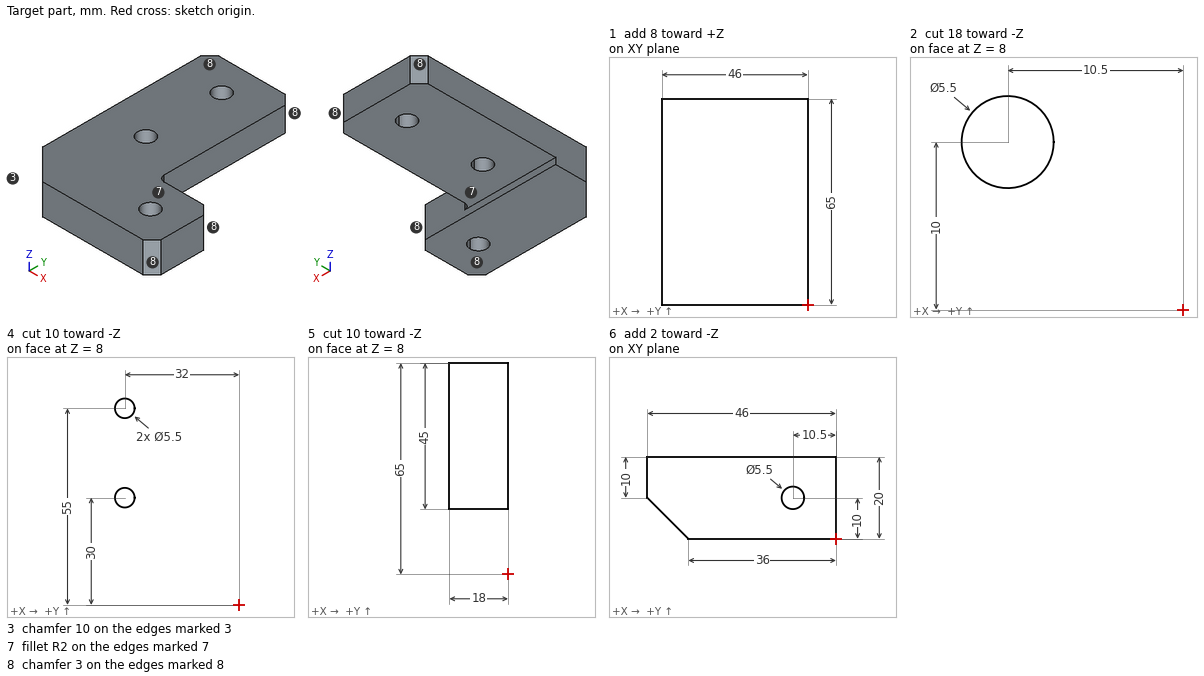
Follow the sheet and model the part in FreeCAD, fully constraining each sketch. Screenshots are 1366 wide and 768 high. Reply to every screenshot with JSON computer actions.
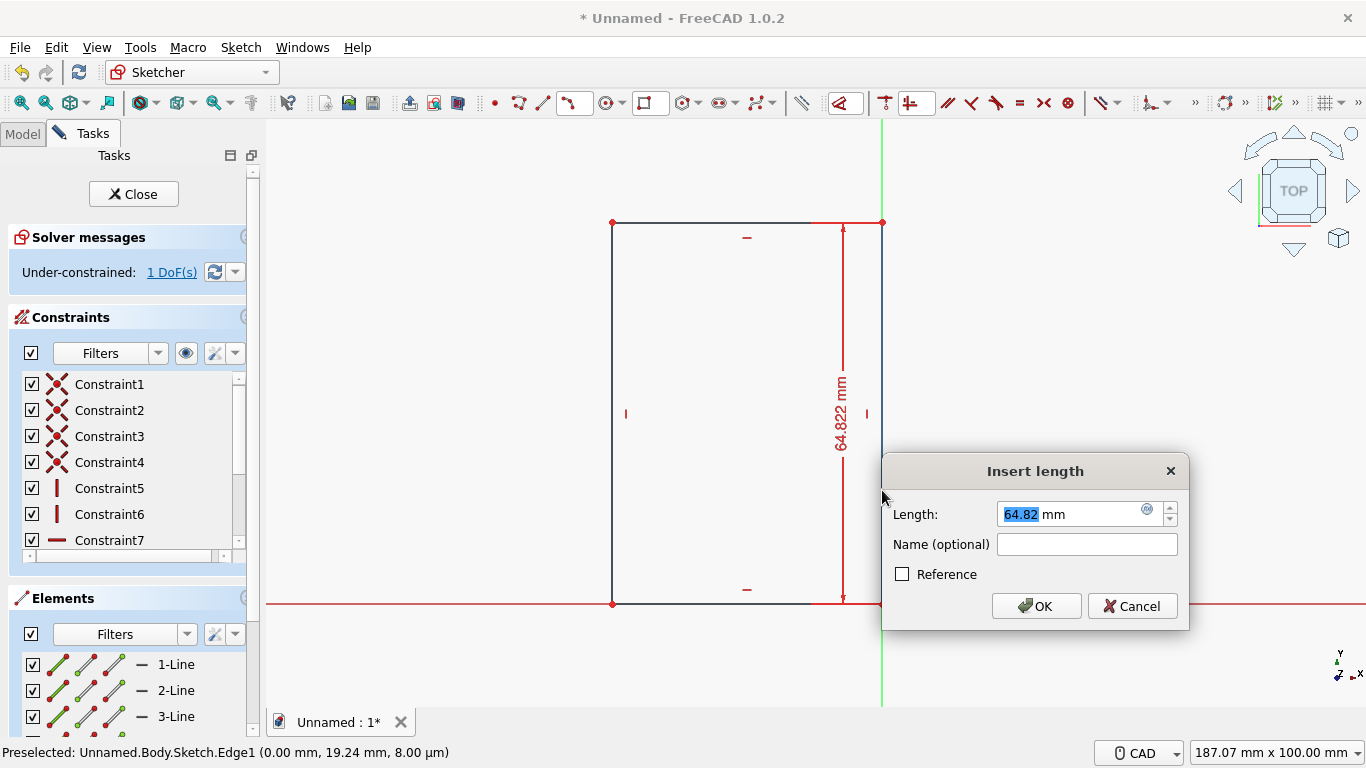
{"action": "type", "text": "65"}
{"action": "key", "text": "Return"}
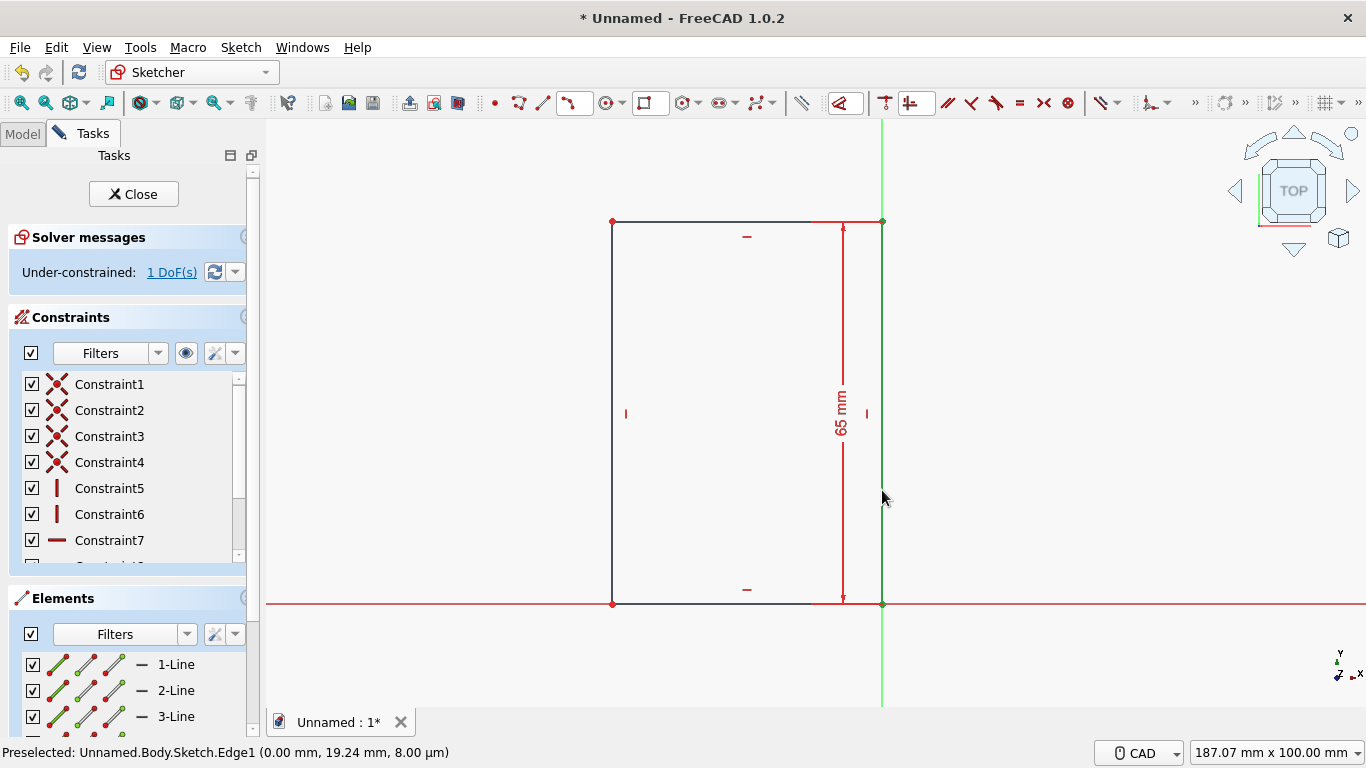
{"action": "left_click", "coordinate": [801, 222]}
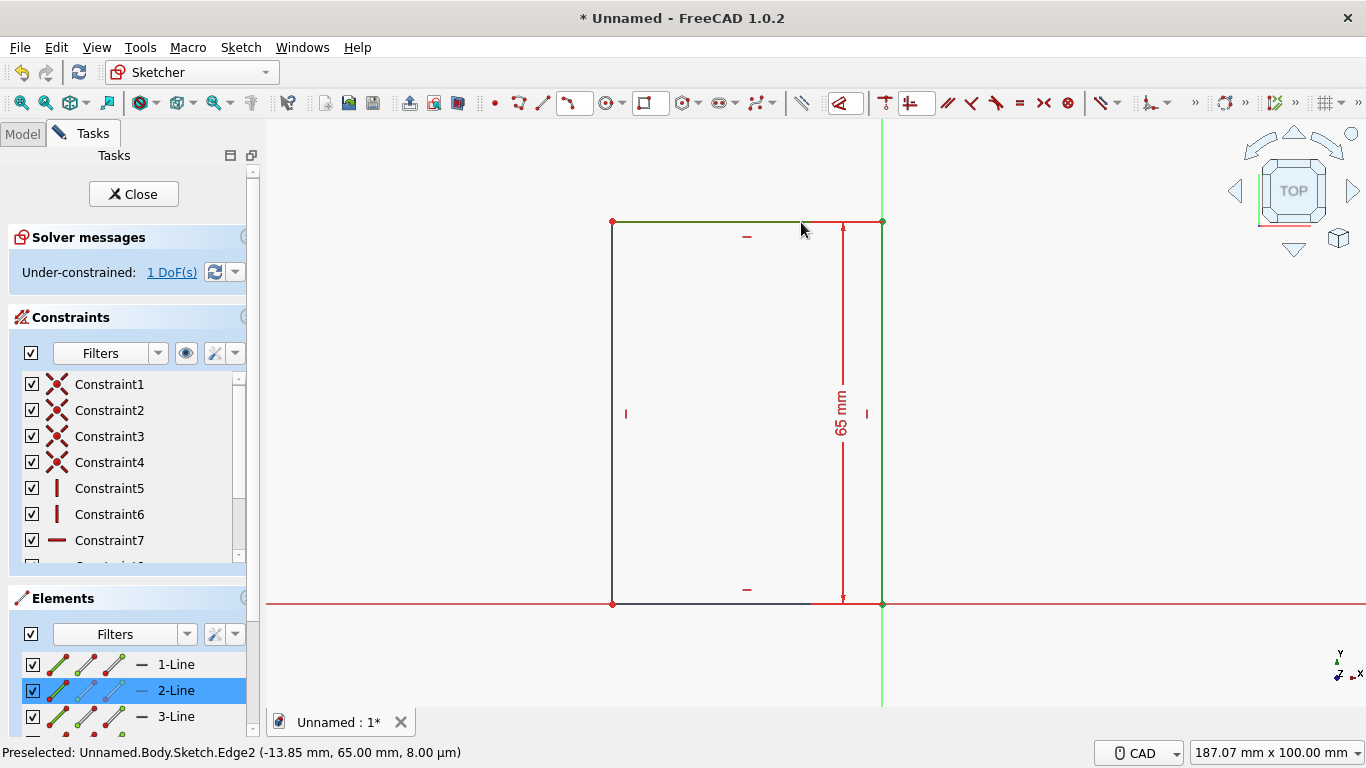
{"action": "key", "text": "l"}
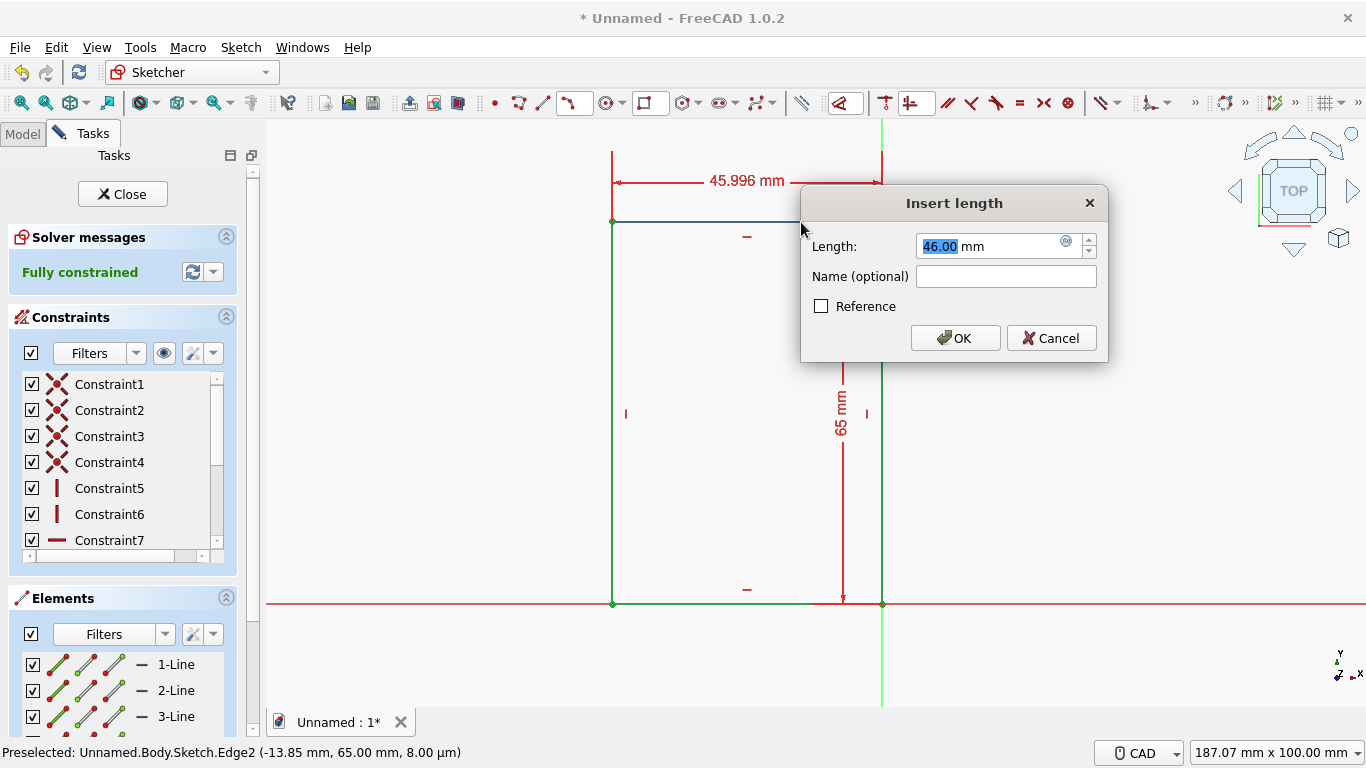
{"action": "type", "text": "46"}
{"action": "key", "text": "Return"}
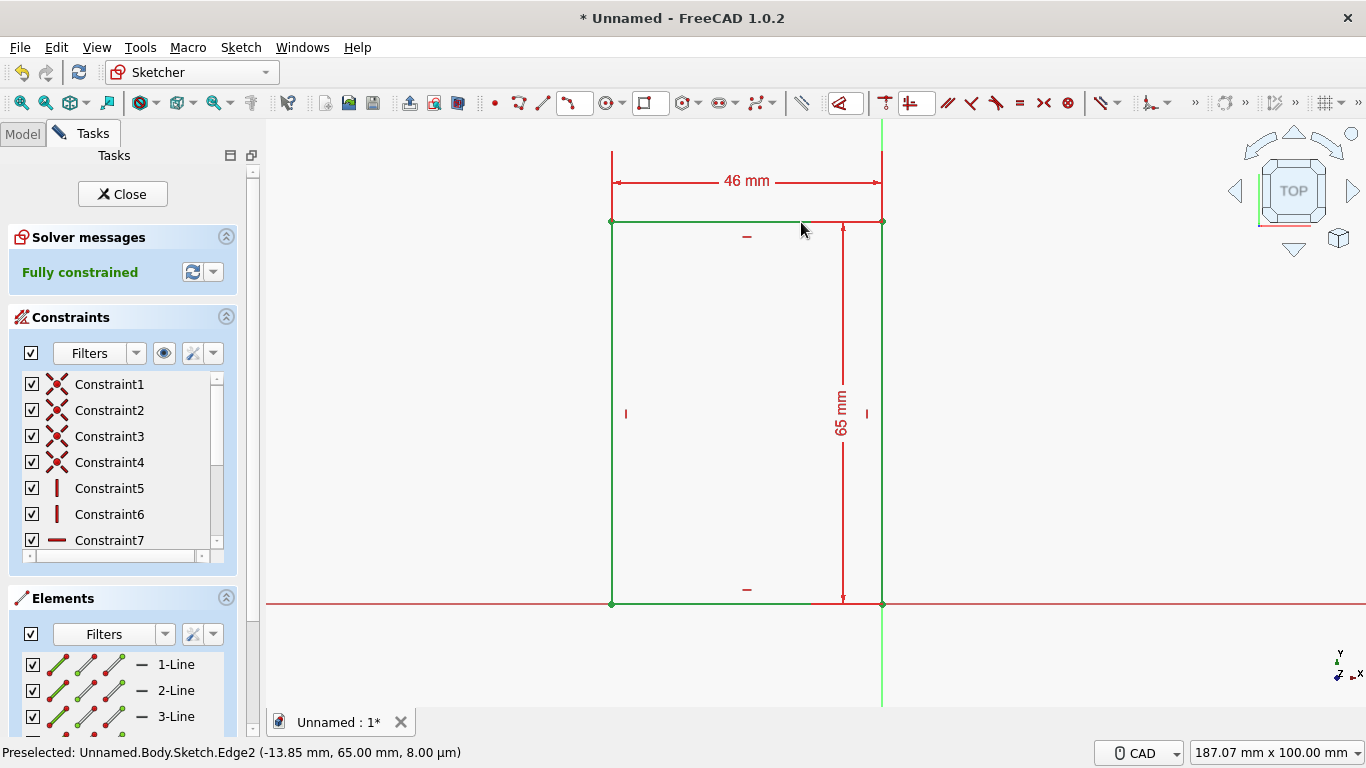
{"action": "left_click", "coordinate": [123, 194]}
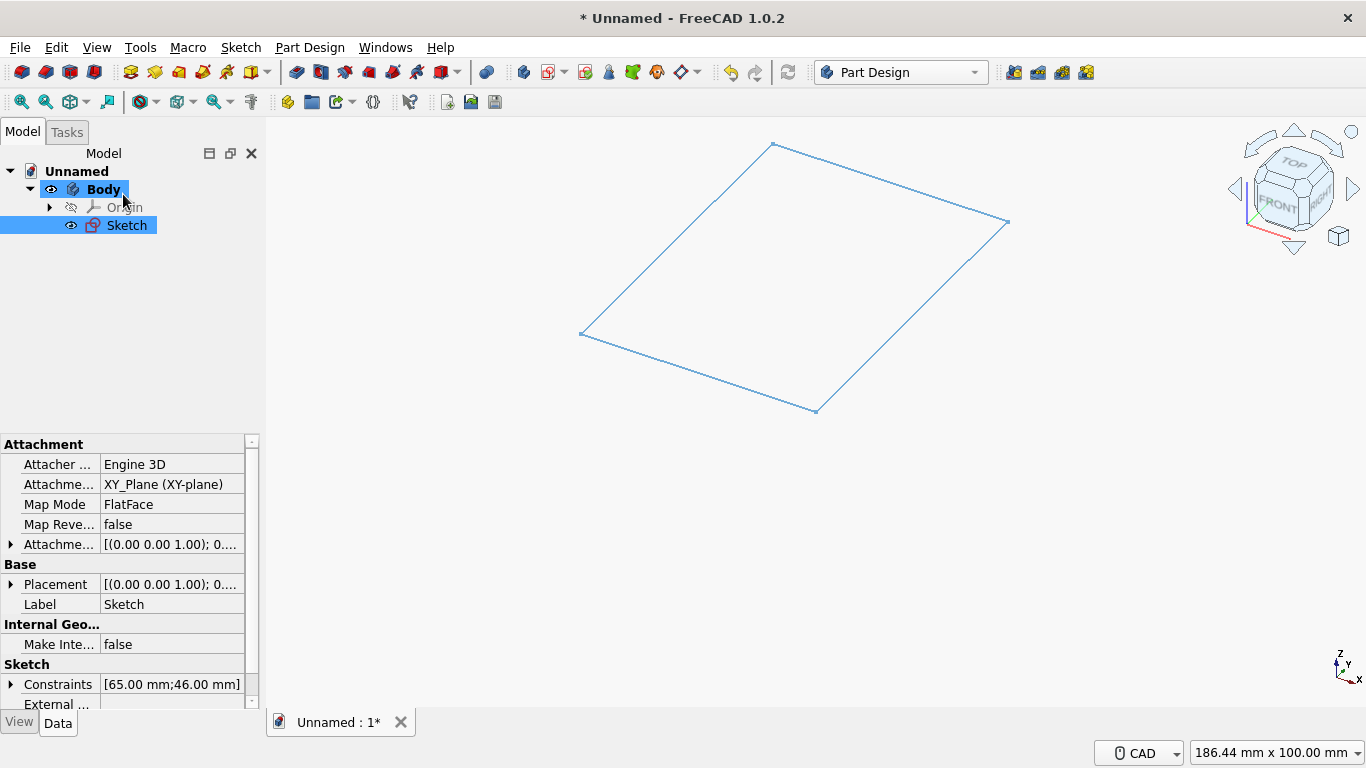
{"action": "left_click", "coordinate": [132, 72]}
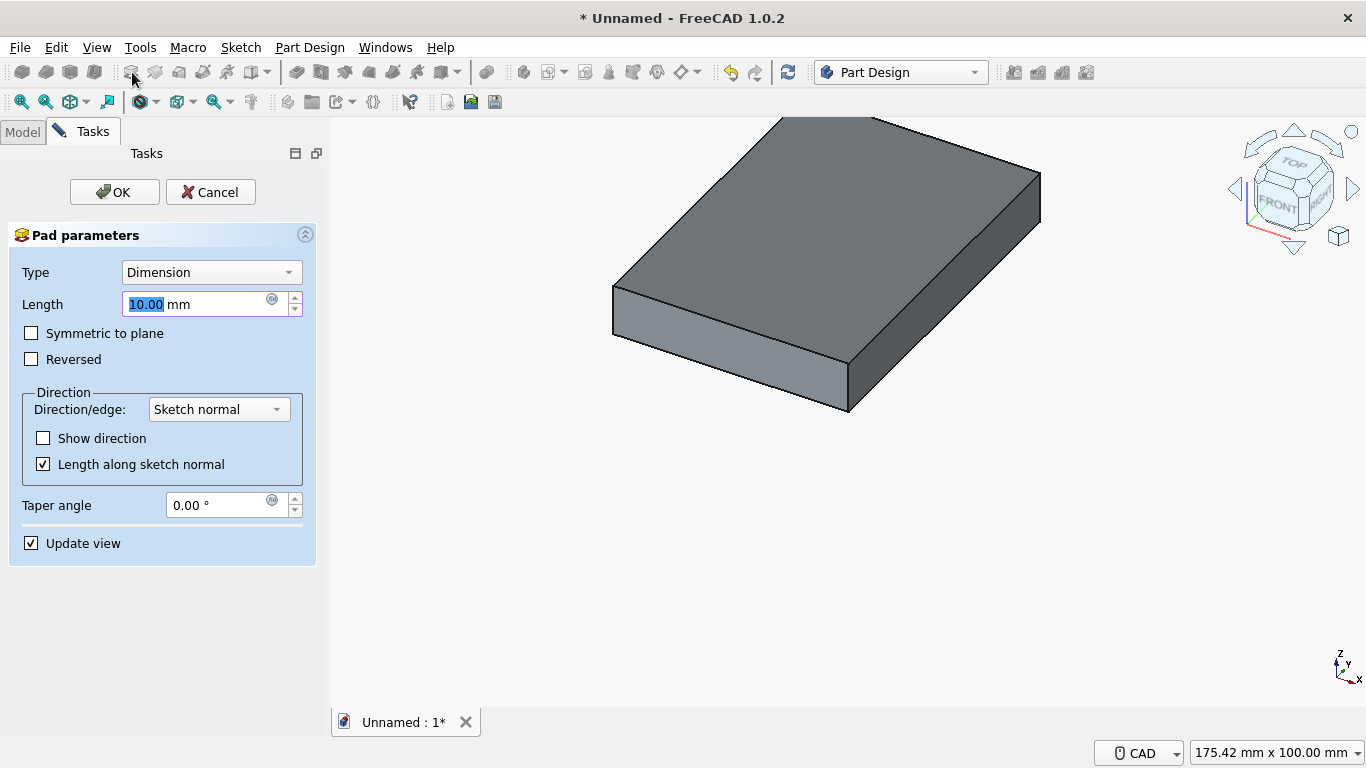
{"action": "type", "text": "8"}
{"action": "key", "text": "Tab"}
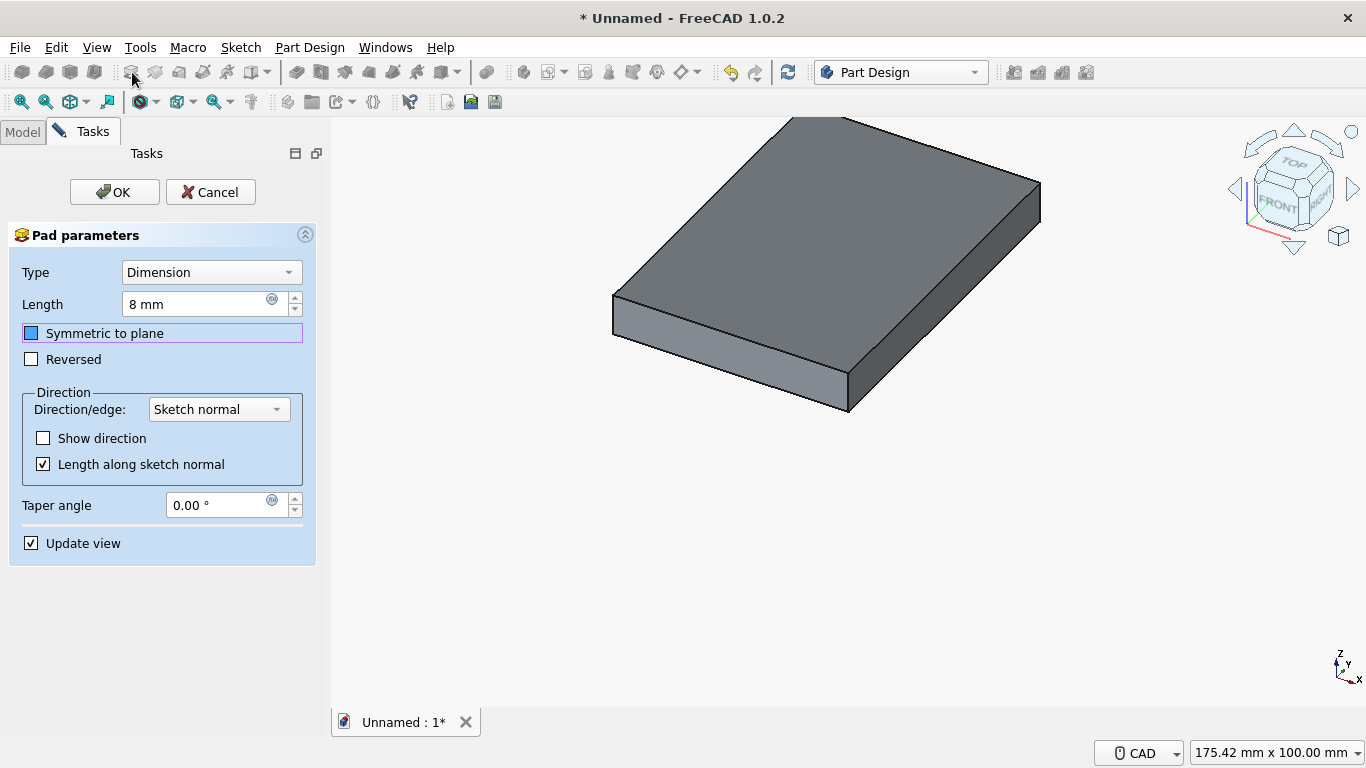
{"action": "left_click", "coordinate": [115, 192]}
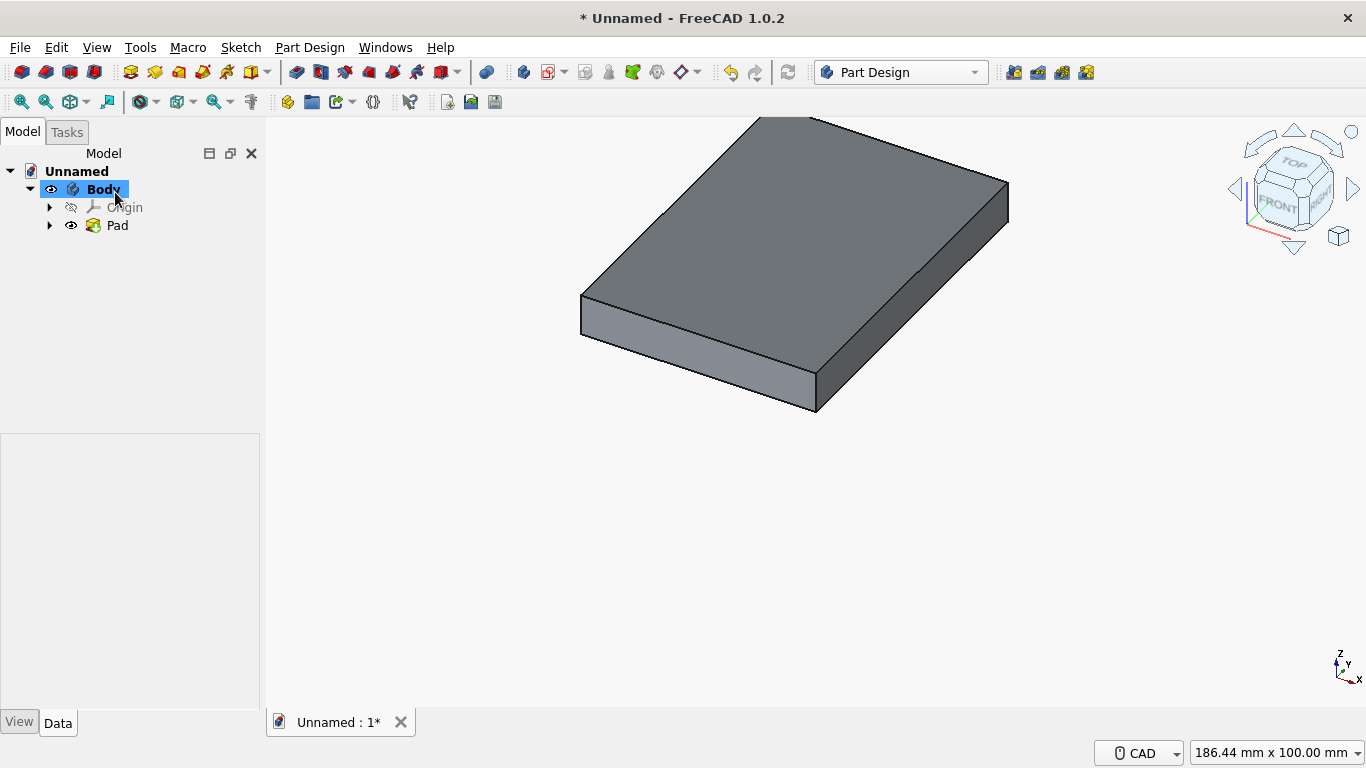
{"action": "key", "text": "v f"}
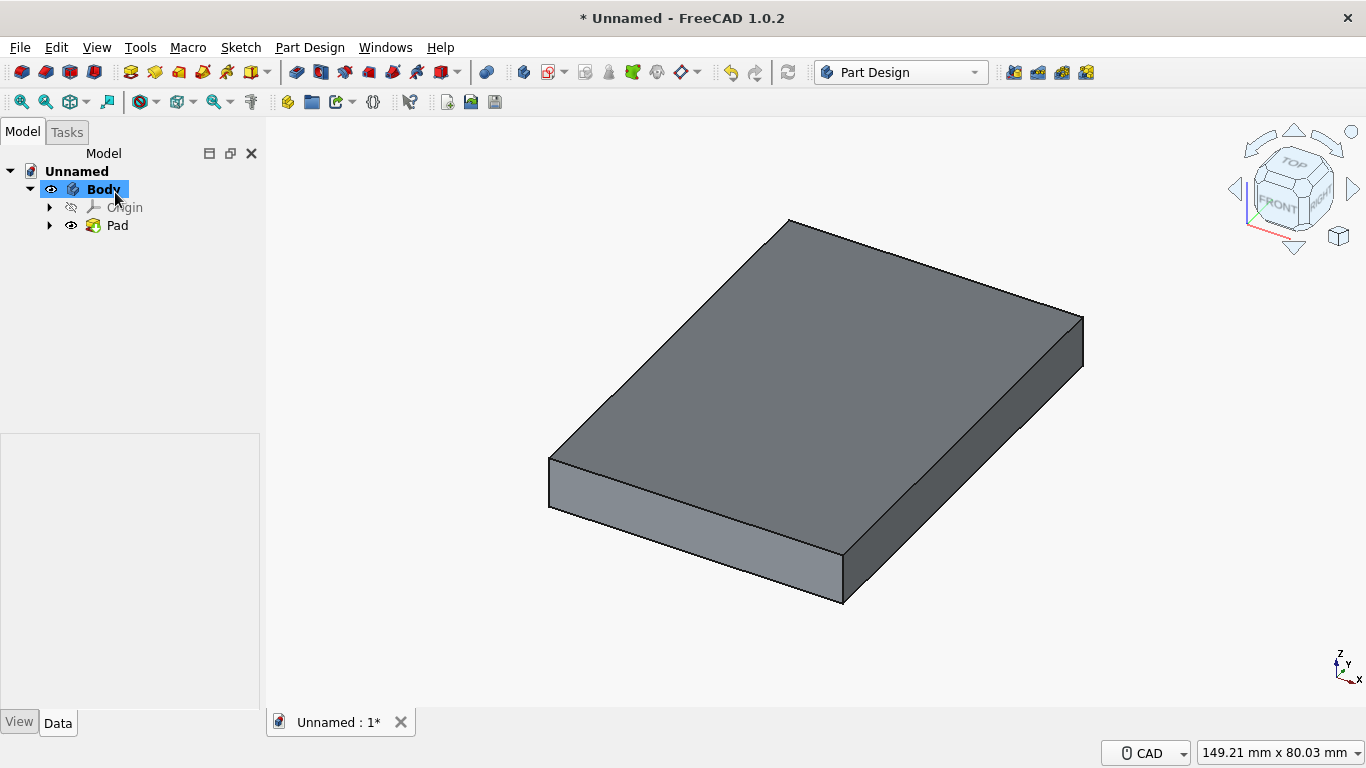
{"action": "left_click", "coordinate": [850, 353]}